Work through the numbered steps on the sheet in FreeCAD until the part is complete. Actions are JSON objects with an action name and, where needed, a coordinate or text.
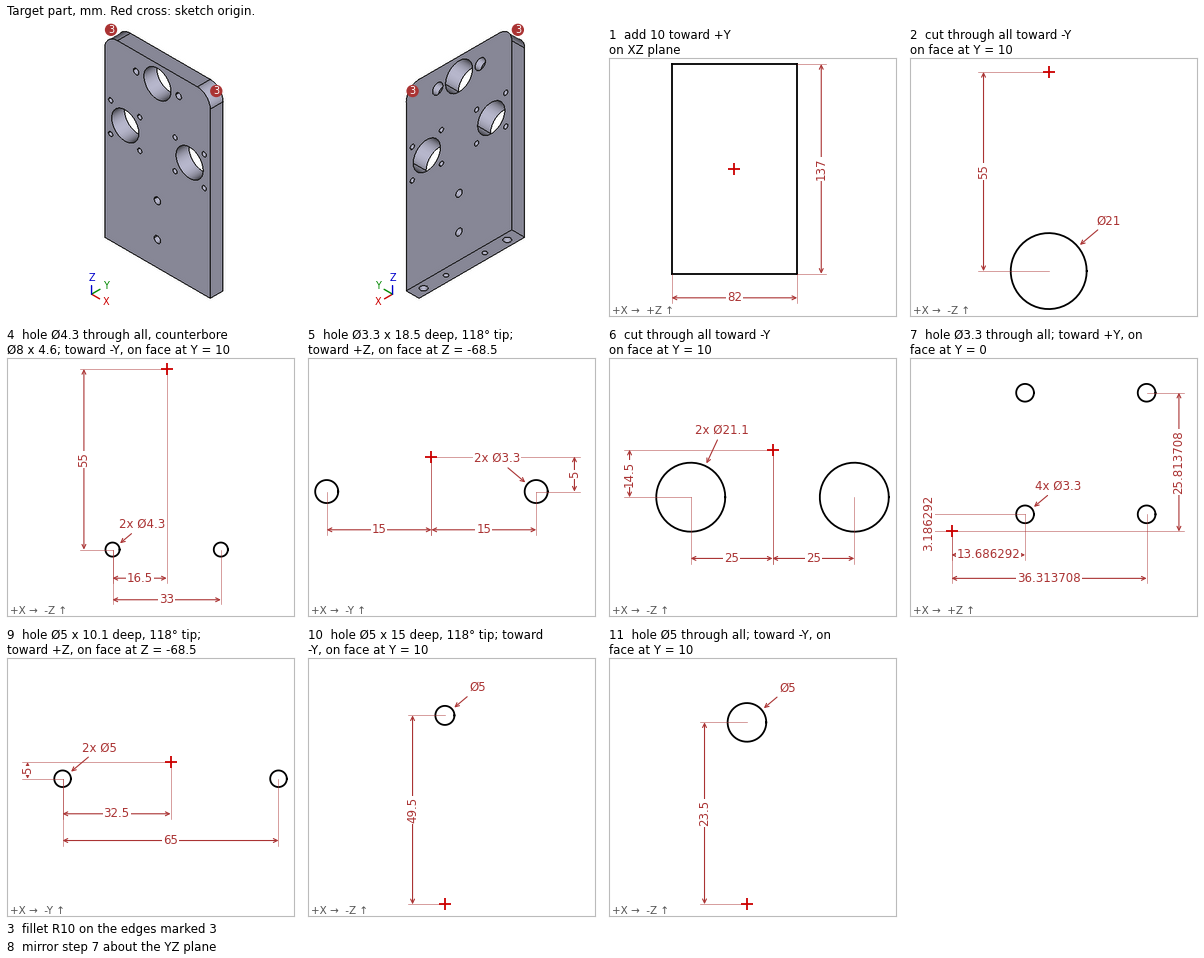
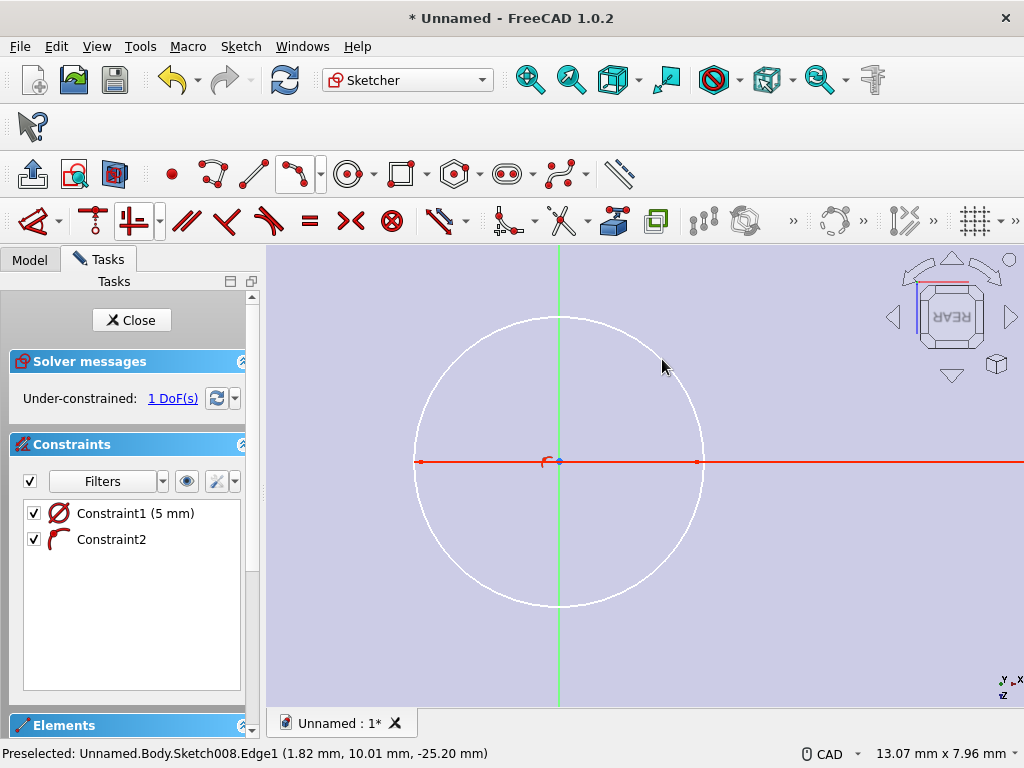
{"action": "left_click", "coordinate": [32, 222]}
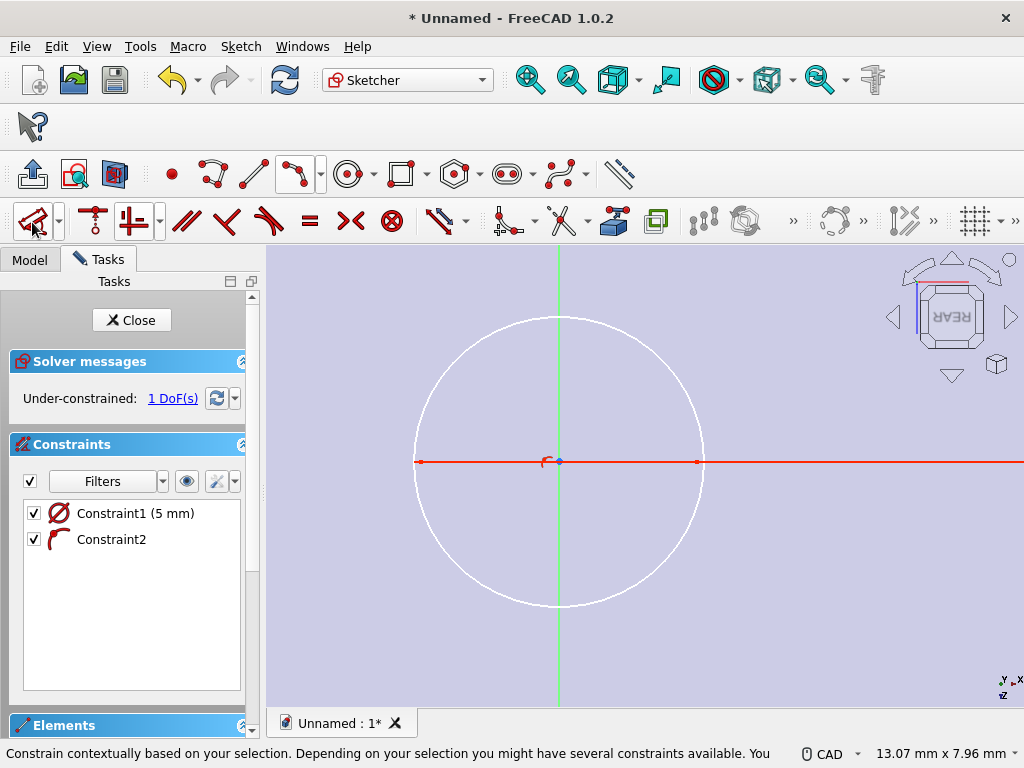
{"action": "left_click", "coordinate": [559, 462]}
{"action": "left_click", "coordinate": [593, 571]}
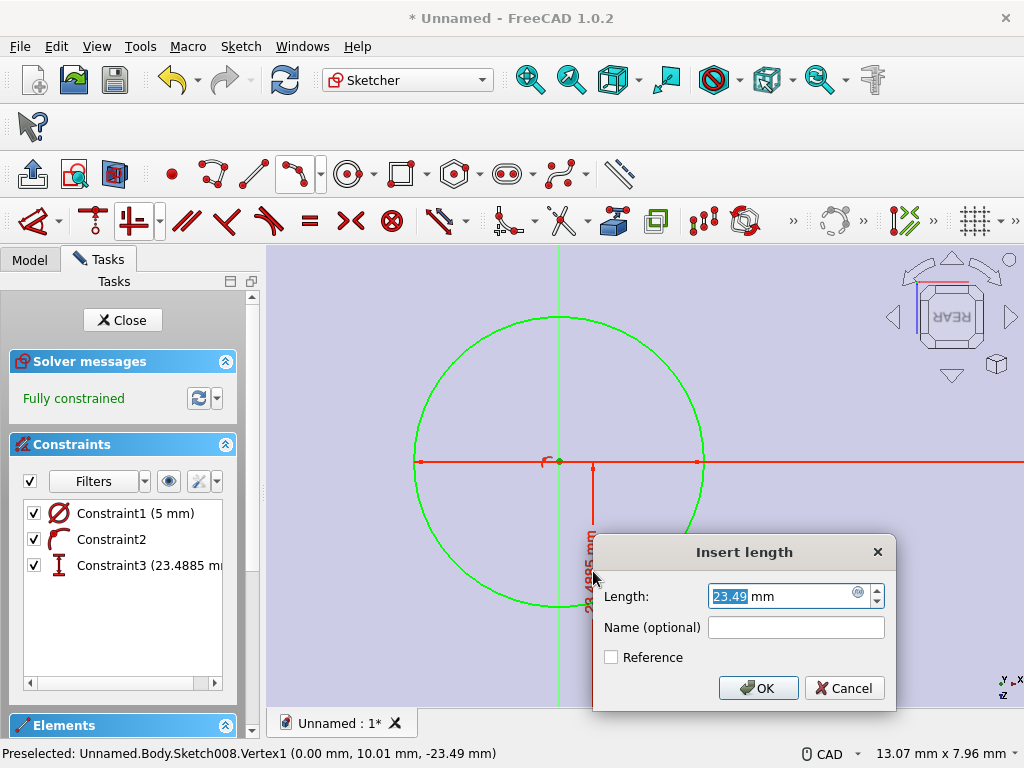
{"action": "type", "text": "23.5"}
{"action": "key", "text": "Return"}
{"action": "key", "text": "Escape"}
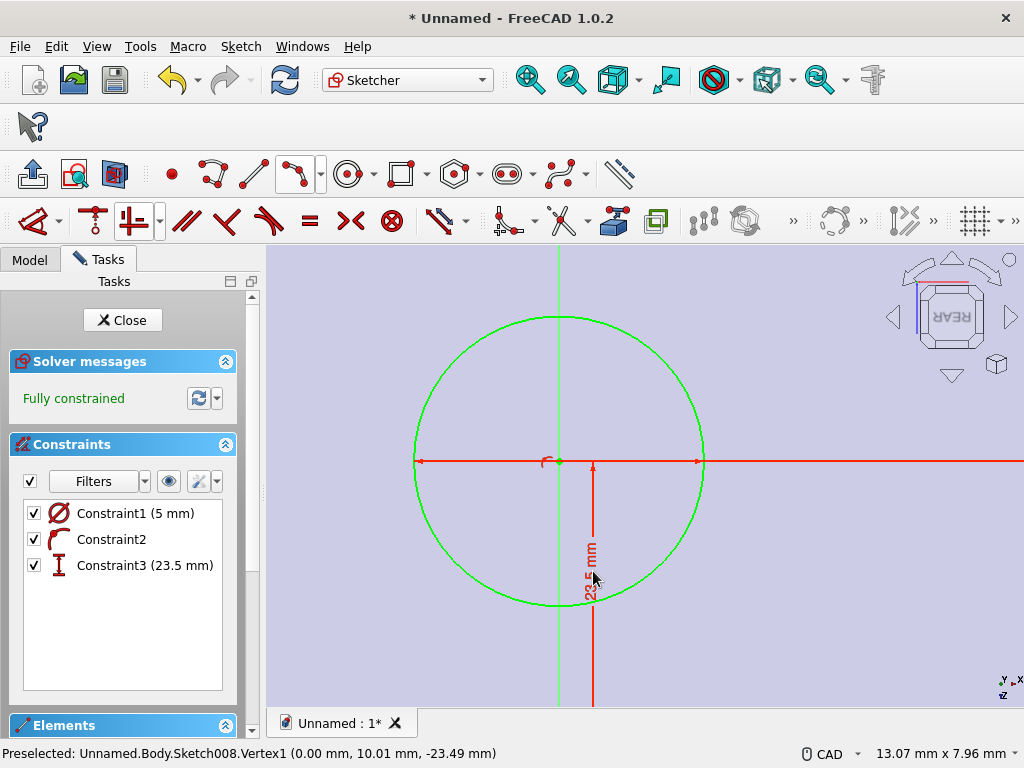
{"action": "left_click", "coordinate": [123, 320]}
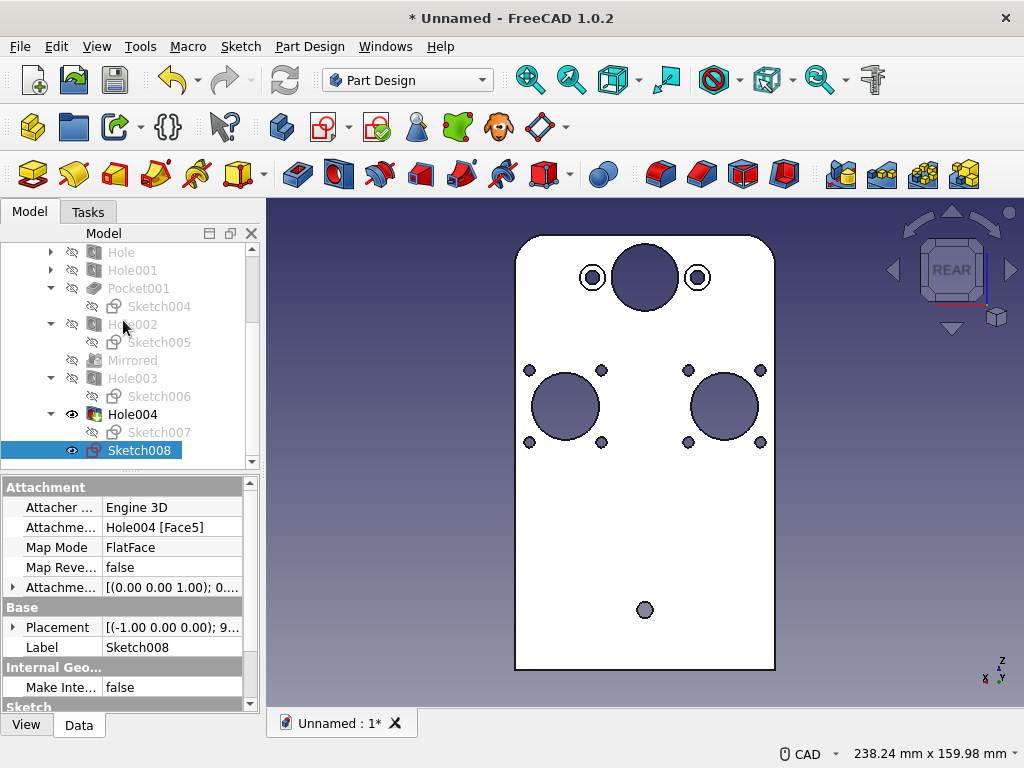
{"action": "left_click", "coordinate": [339, 174]}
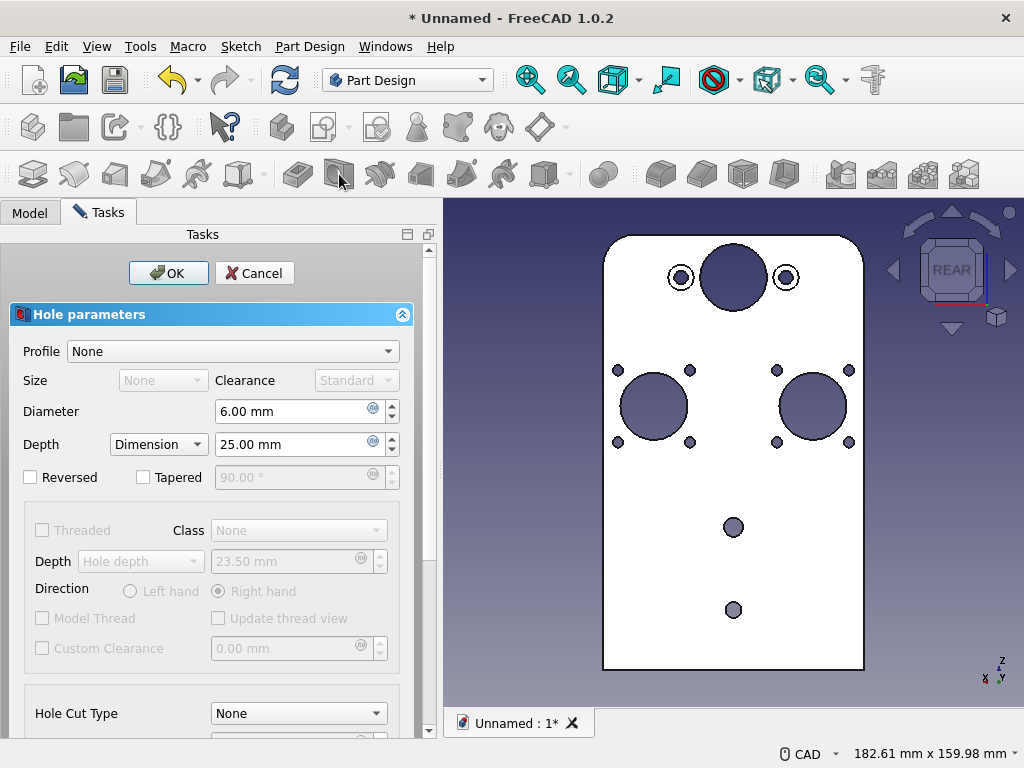
{"action": "triple_click", "coordinate": [300, 412]}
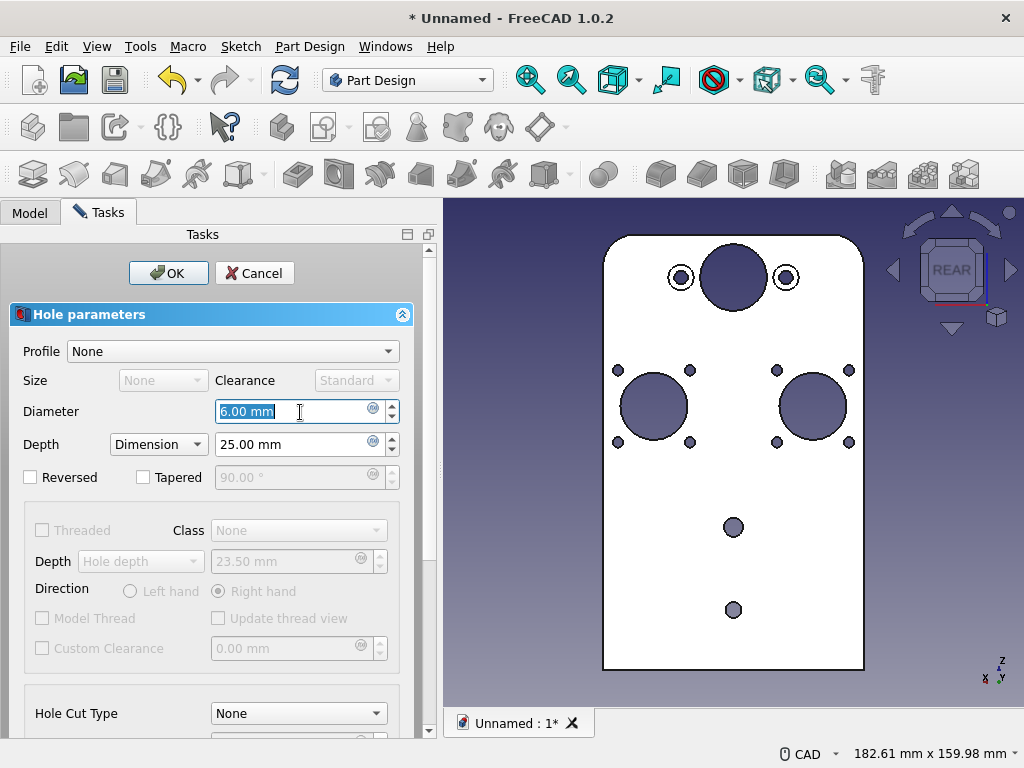
{"action": "type", "text": "5"}
{"action": "key", "text": "Tab"}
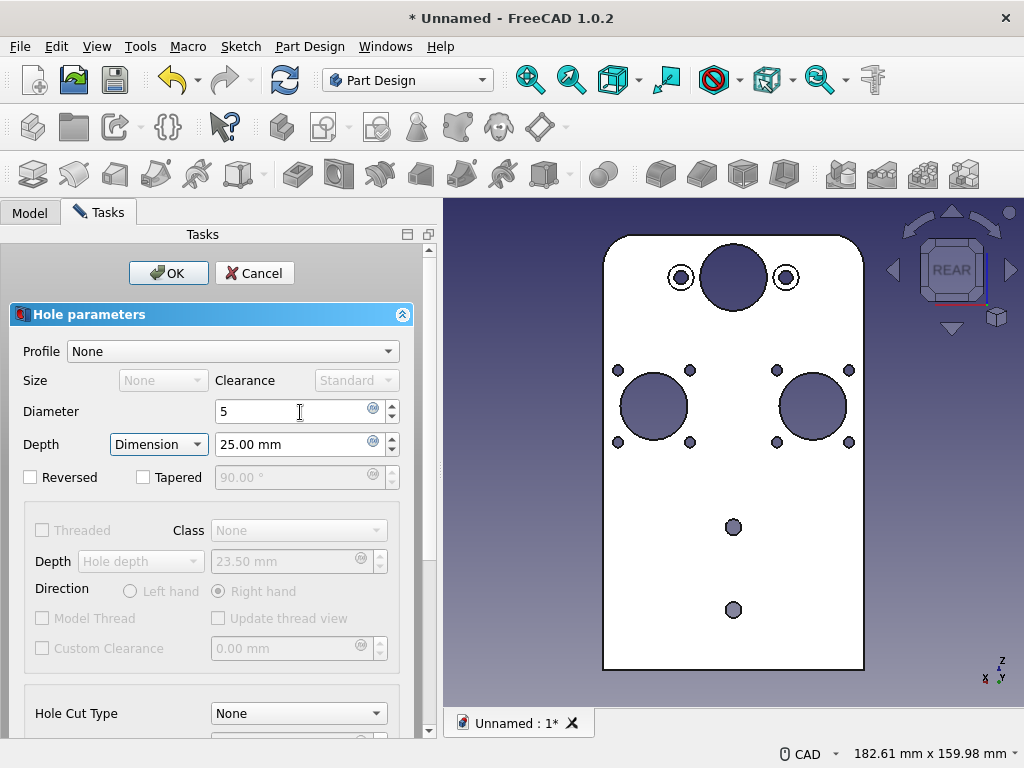
{"action": "left_click", "coordinate": [160, 444]}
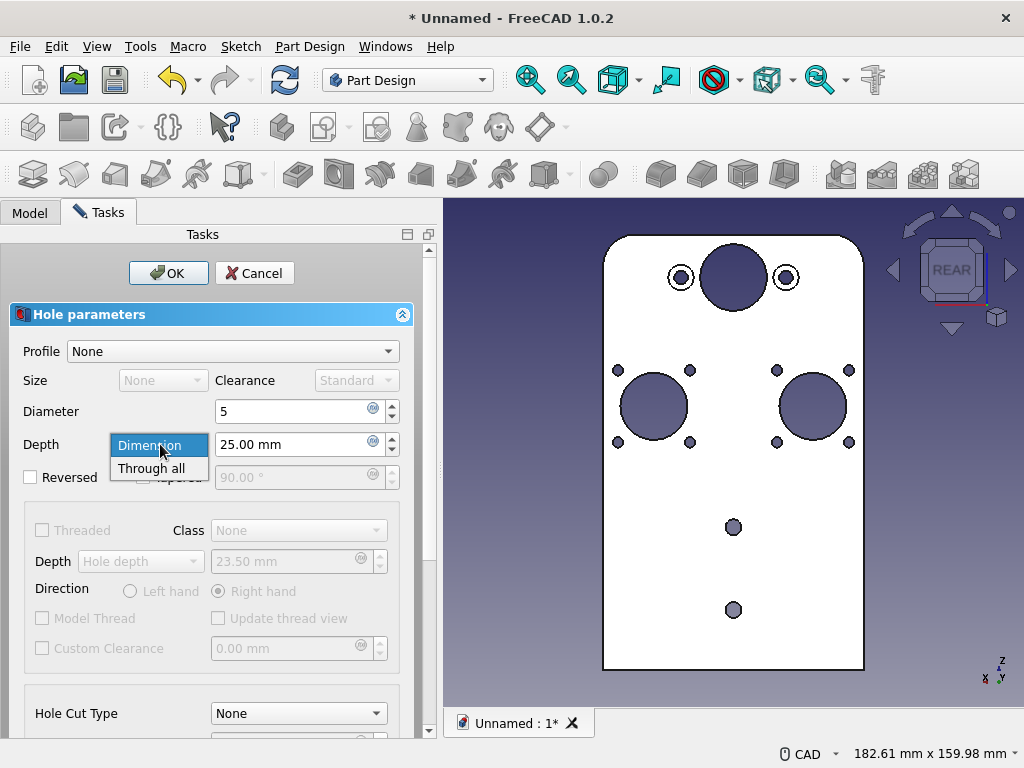
{"action": "left_click", "coordinate": [158, 468]}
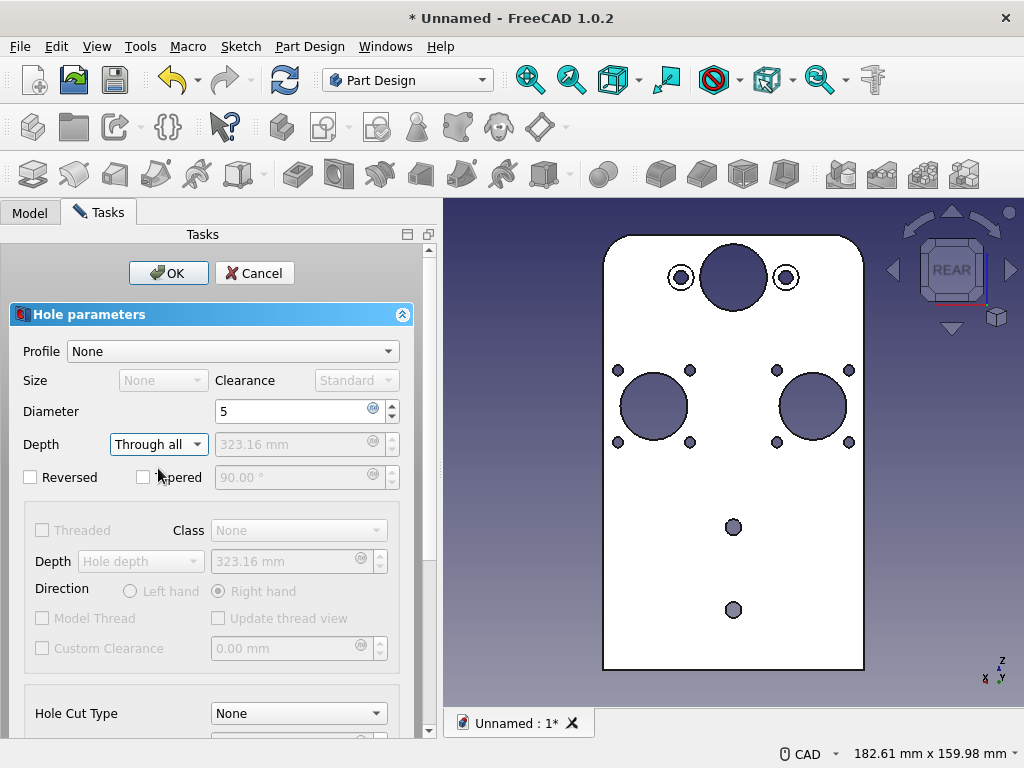
{"action": "left_click", "coordinate": [169, 273]}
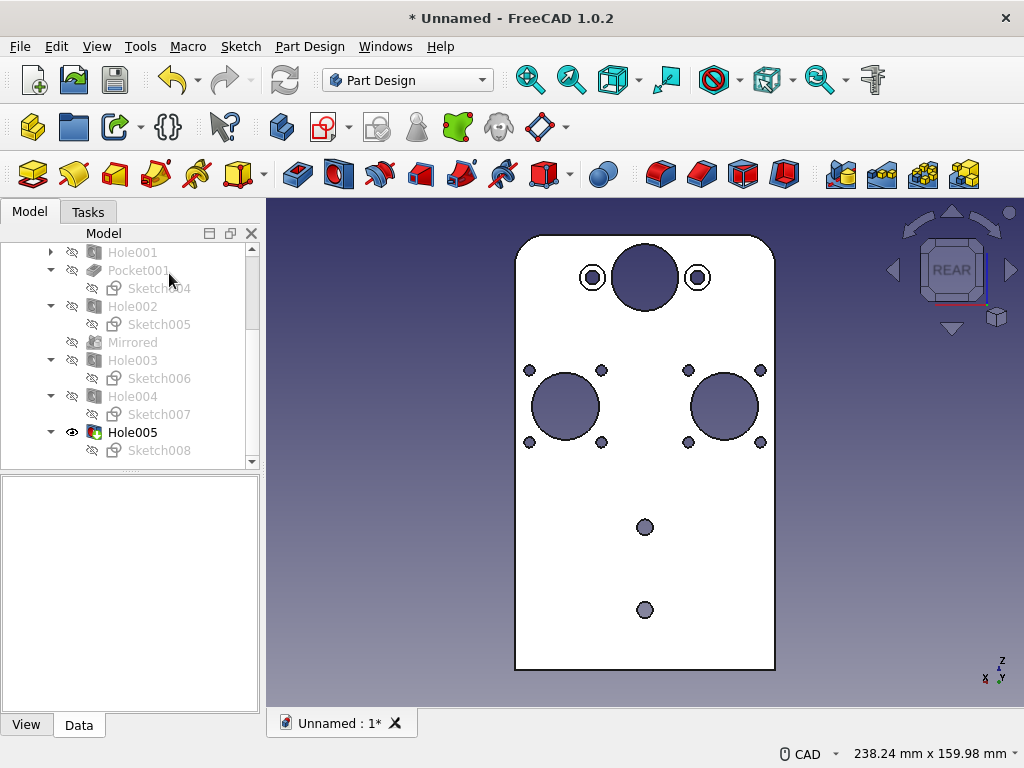
{"action": "key", "text": "0"}